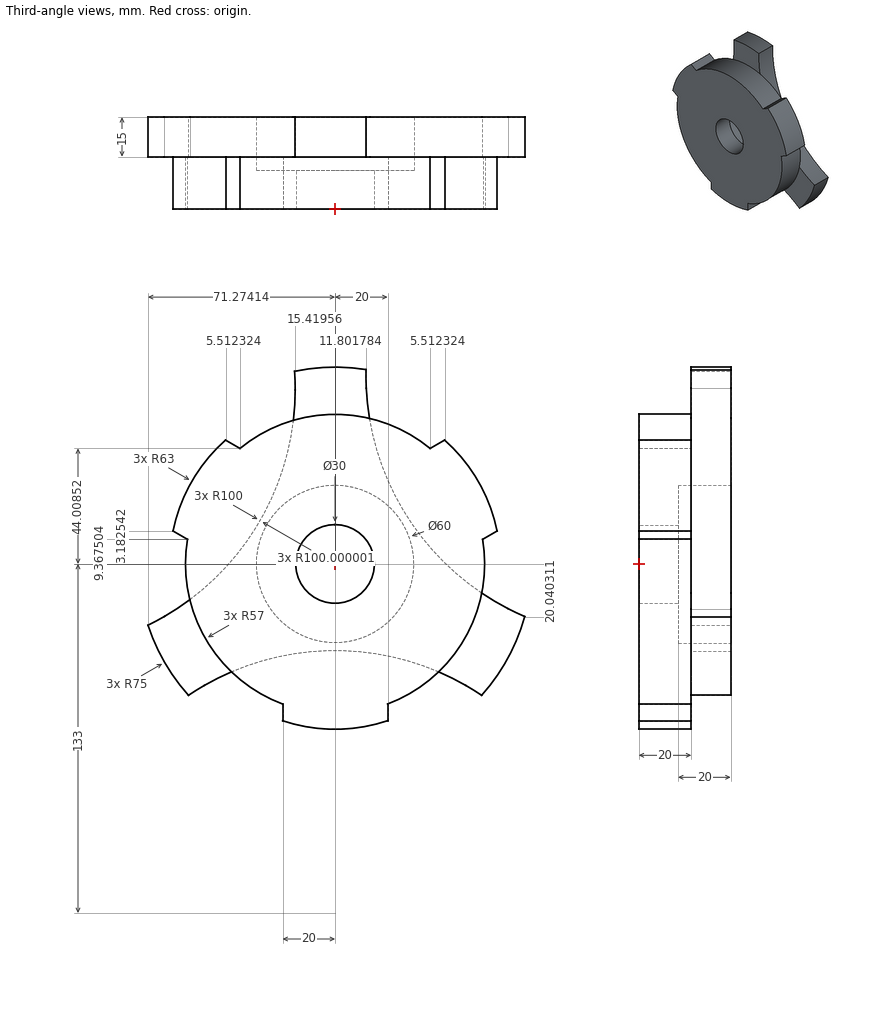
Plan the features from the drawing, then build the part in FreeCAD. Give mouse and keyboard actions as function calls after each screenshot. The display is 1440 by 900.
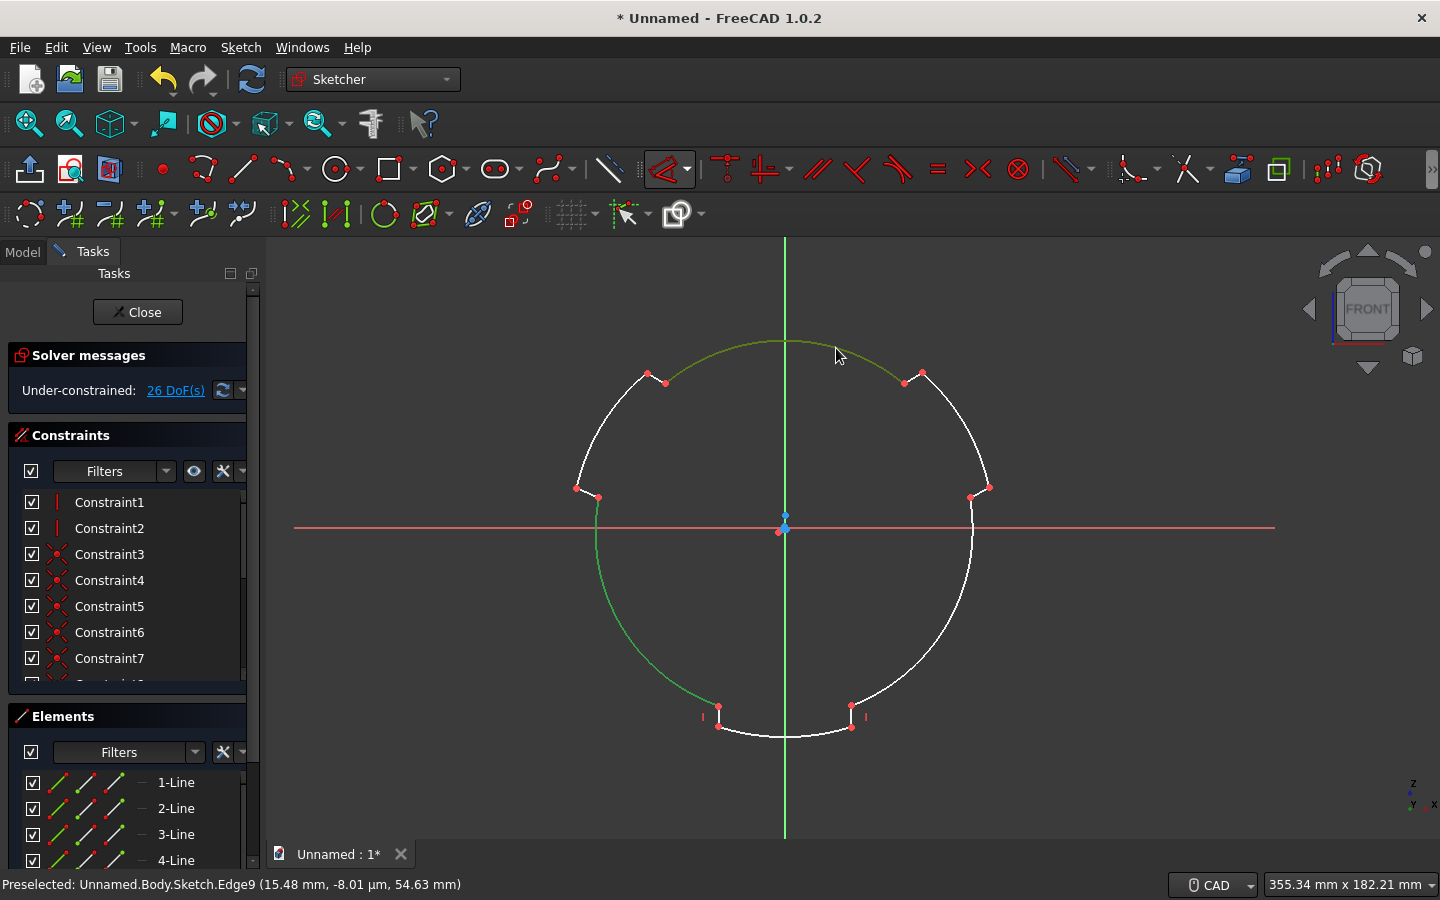
click(726, 170)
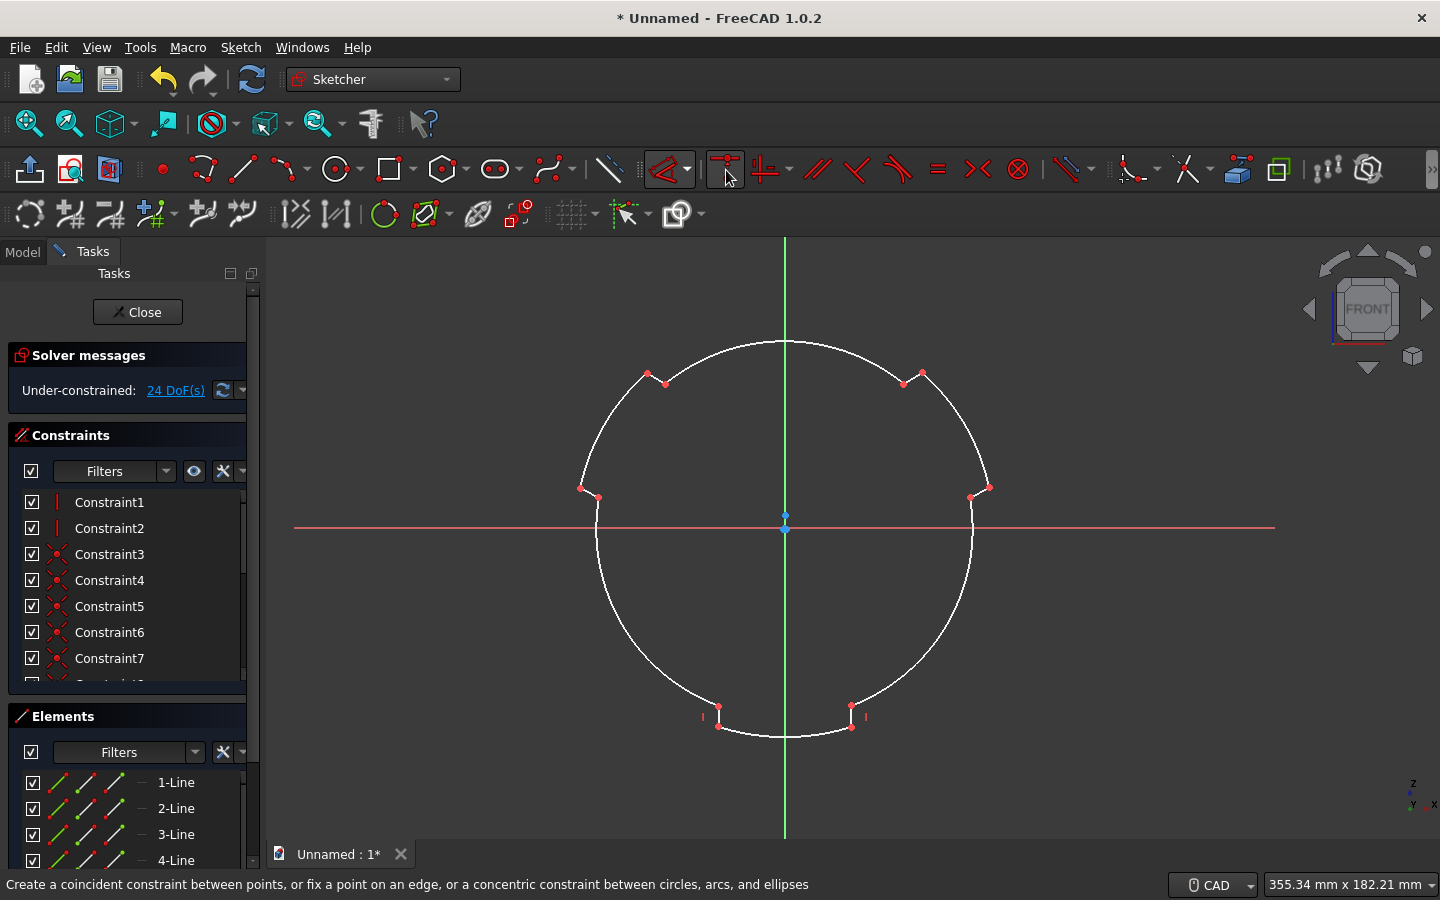
click(602, 576)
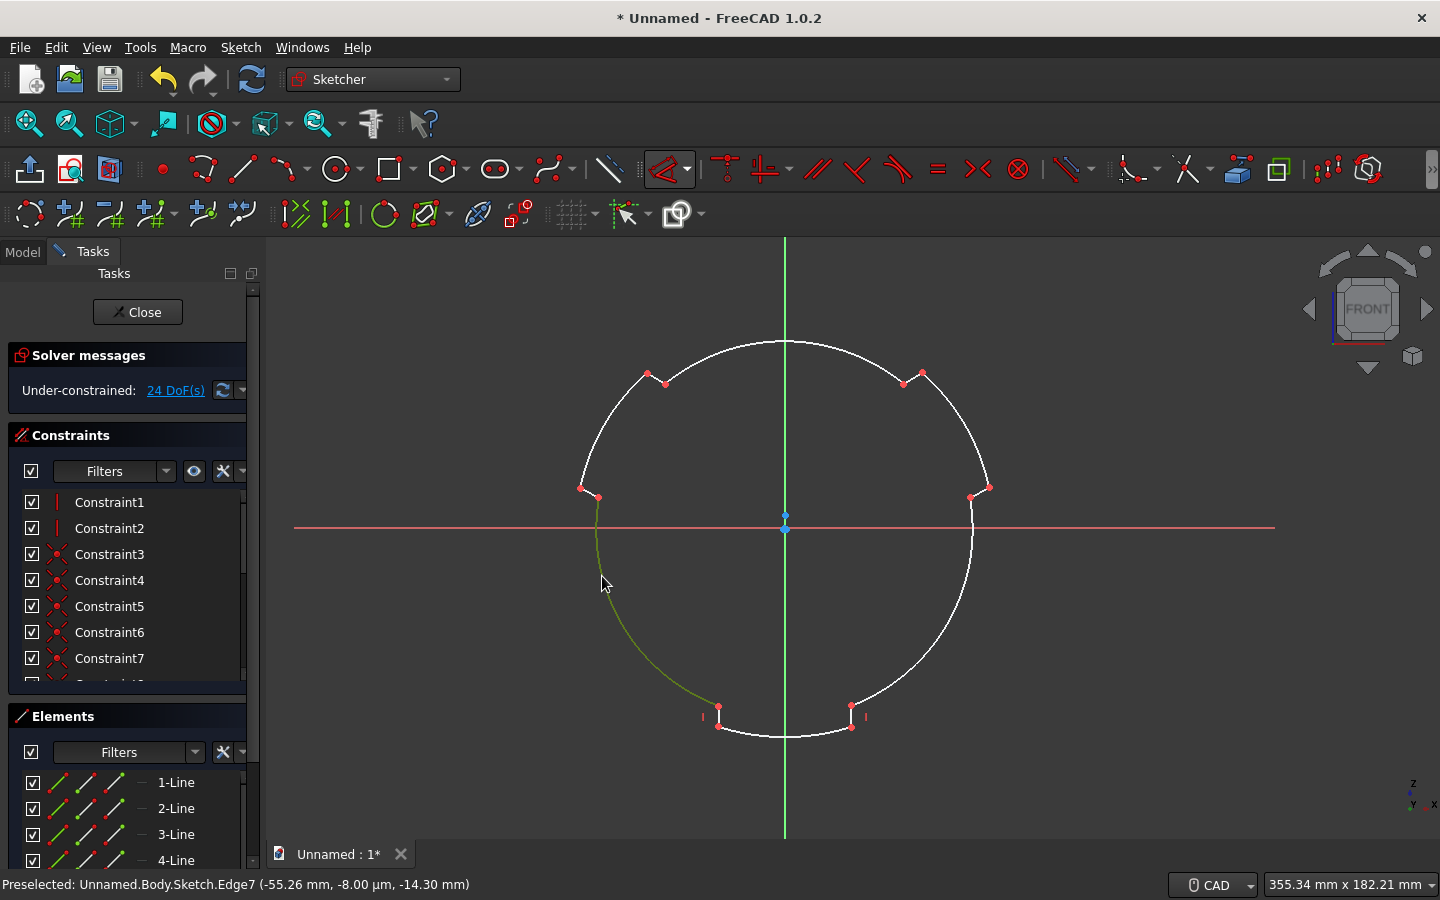
click(977, 449)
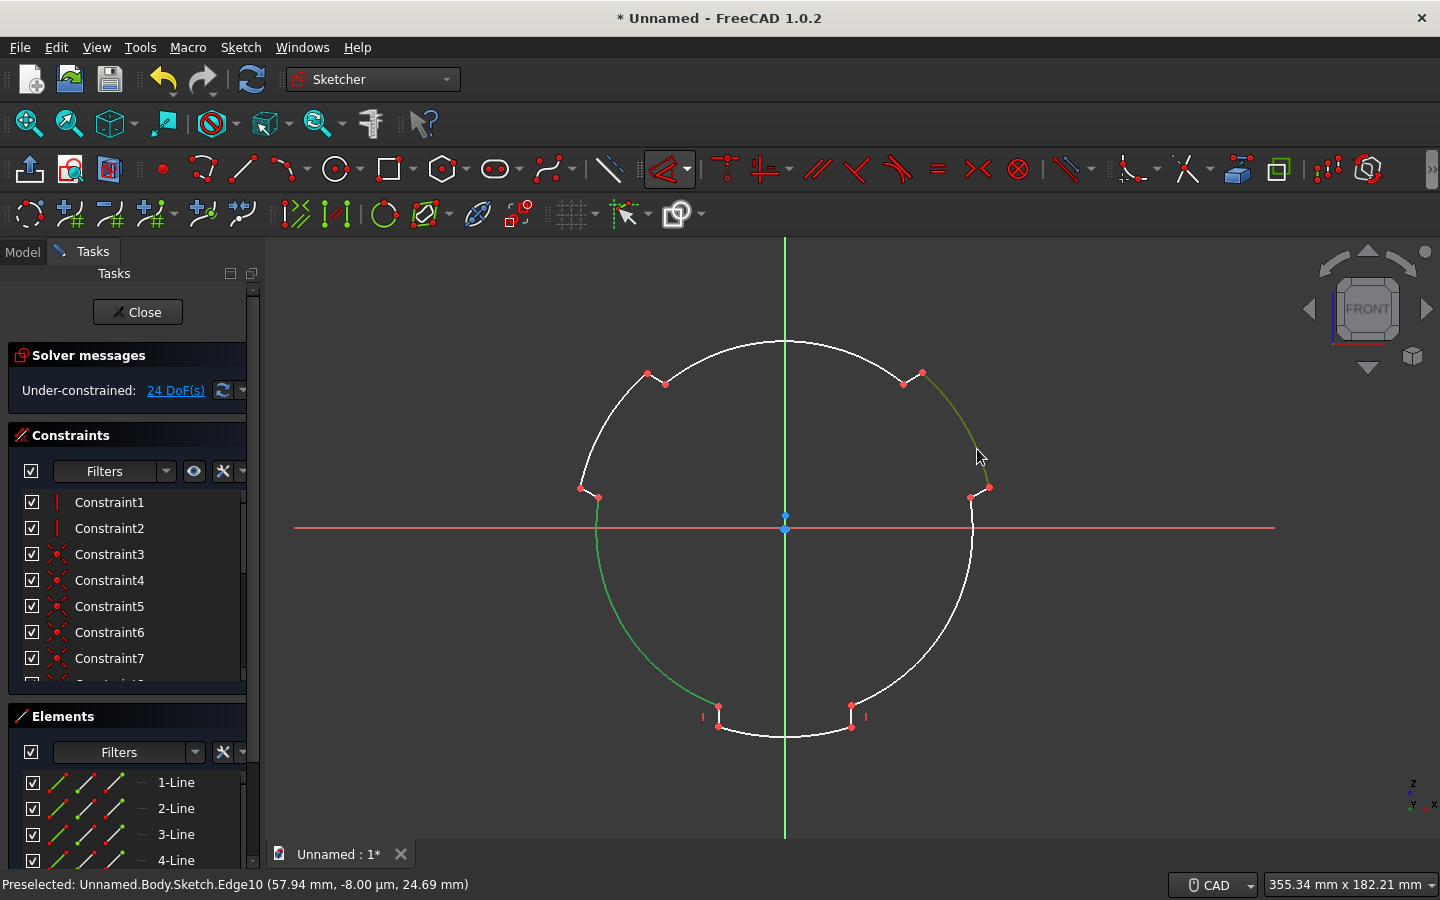
key(c)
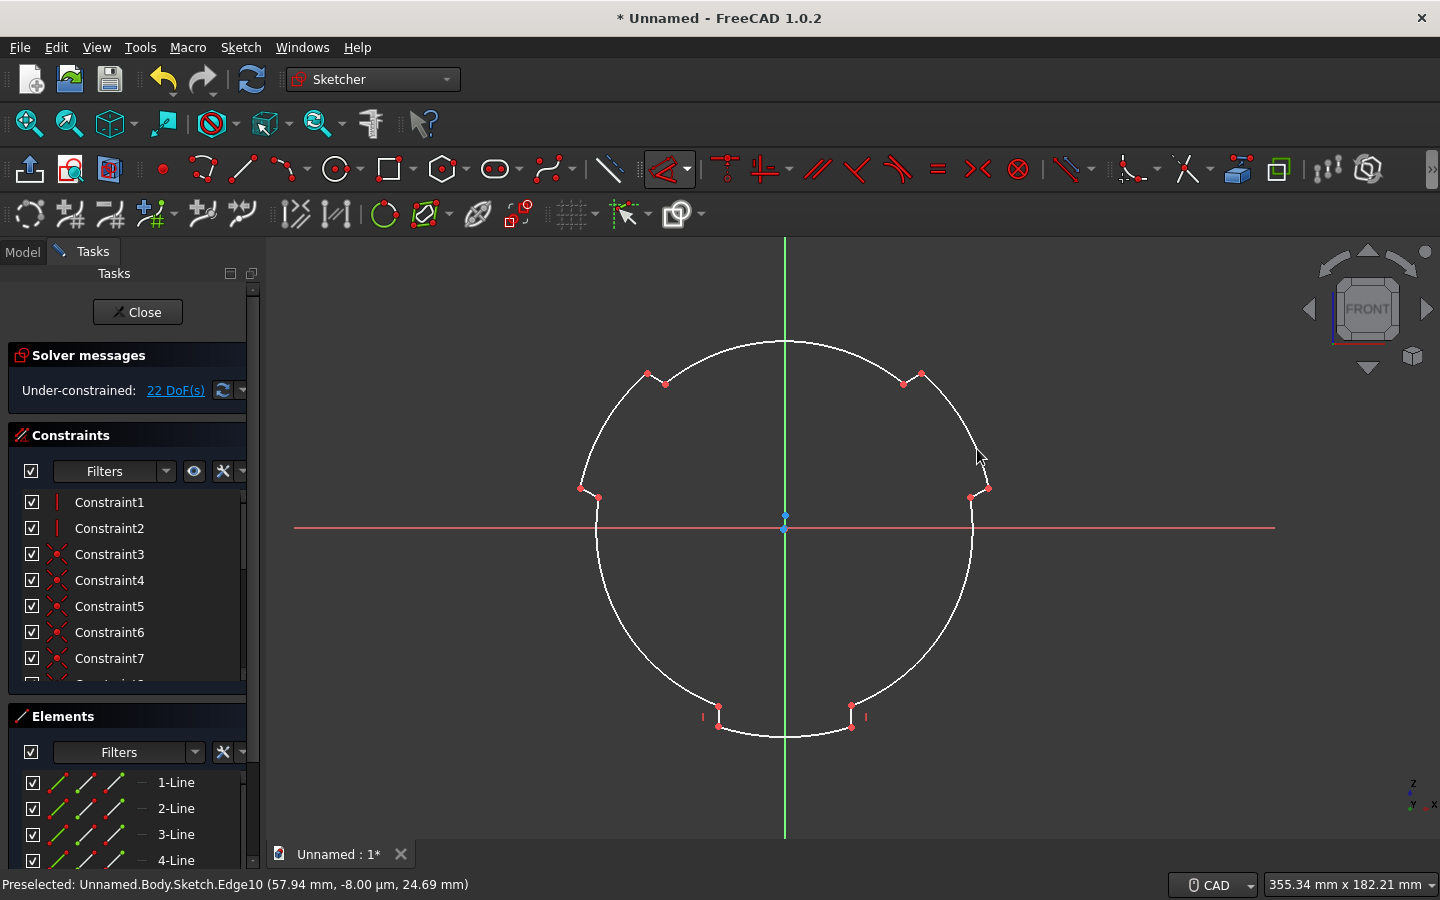
click(602, 576)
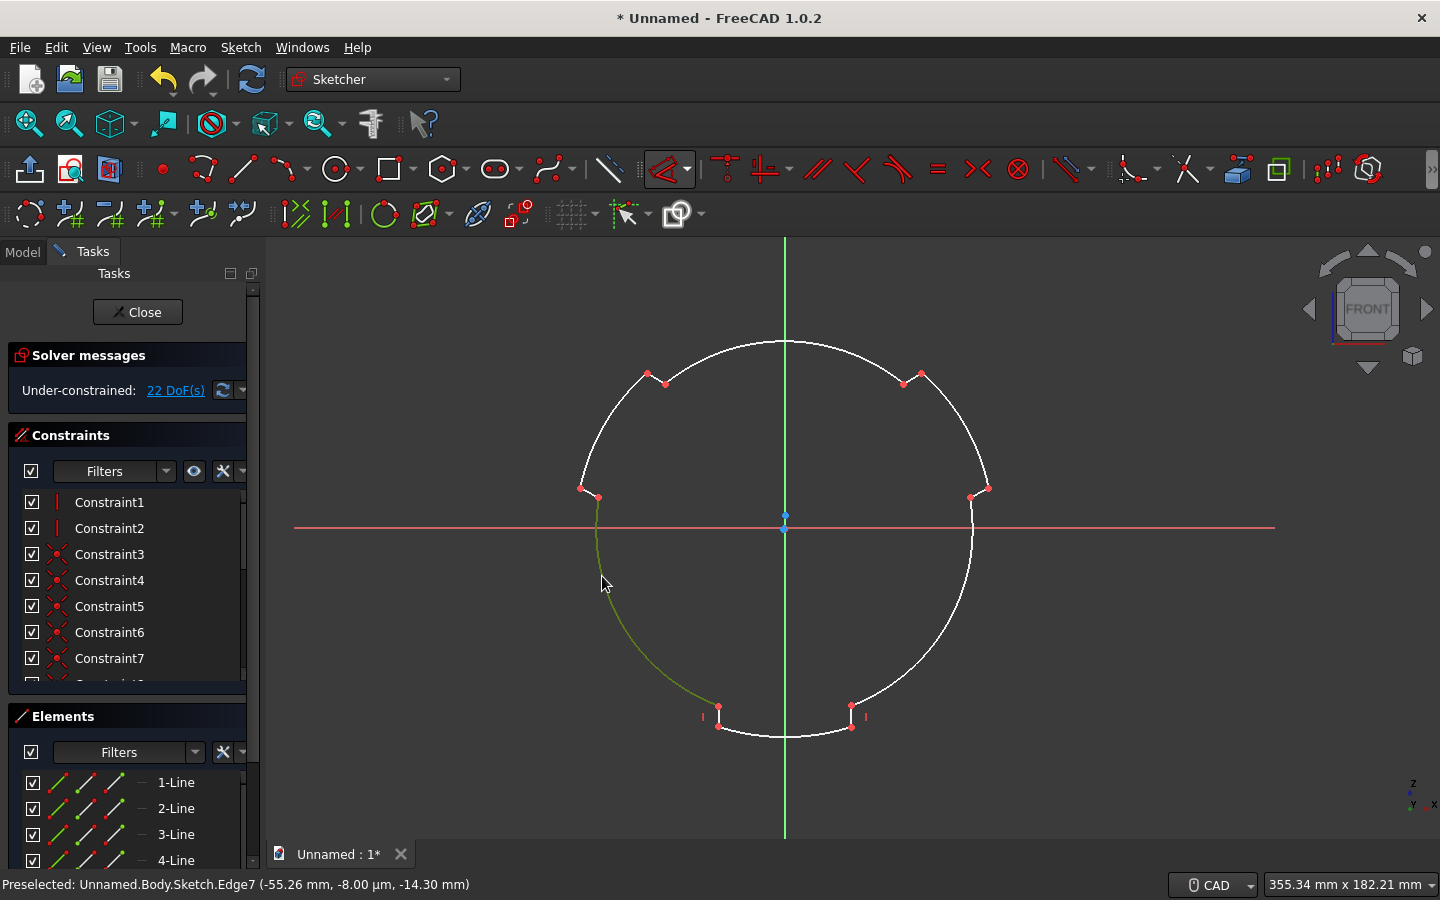
click(916, 664)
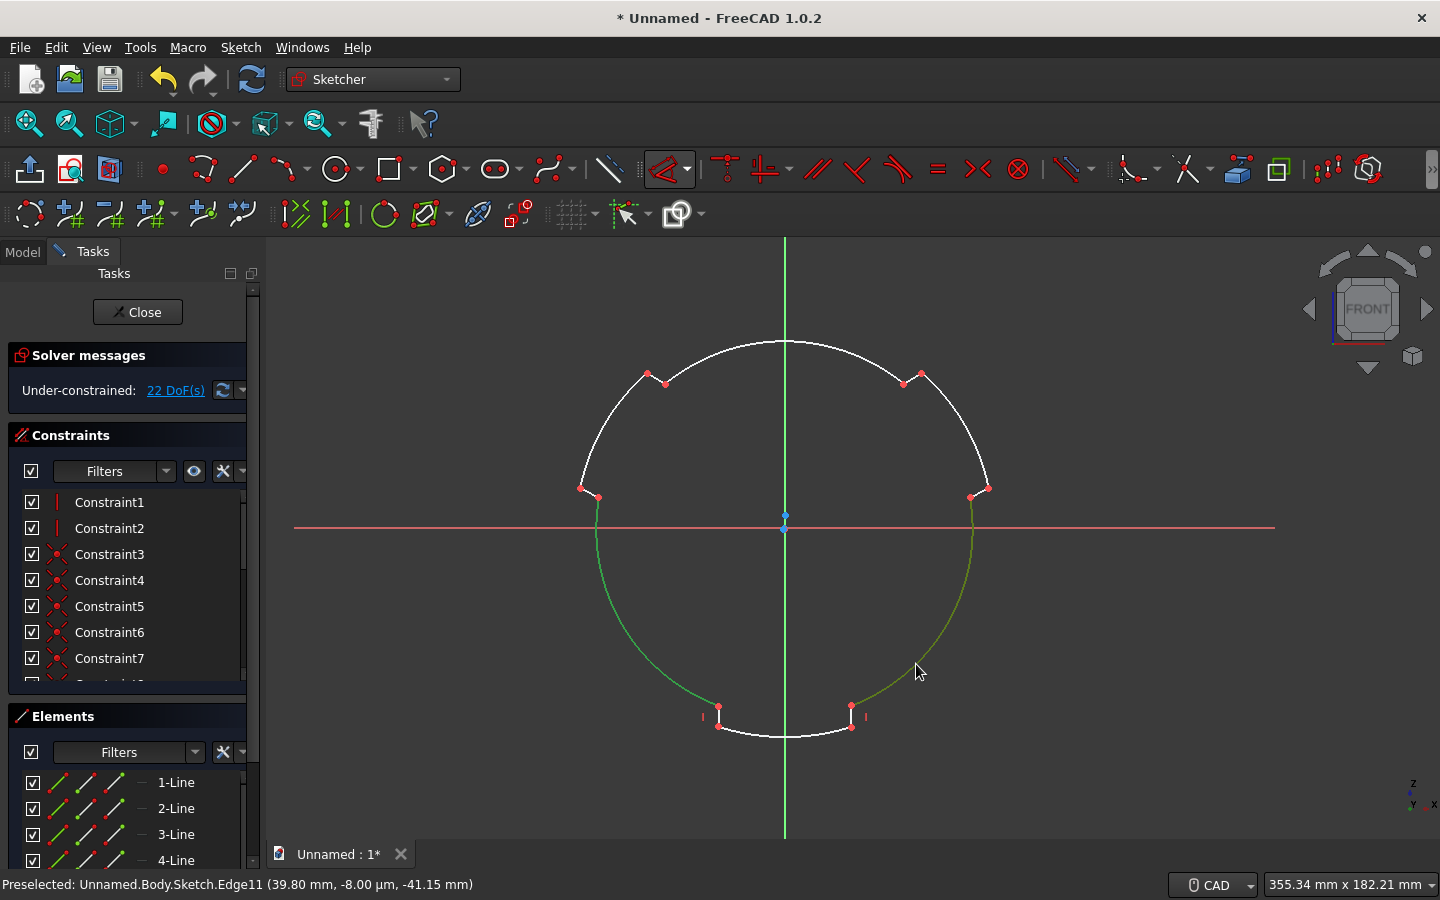
click(726, 170)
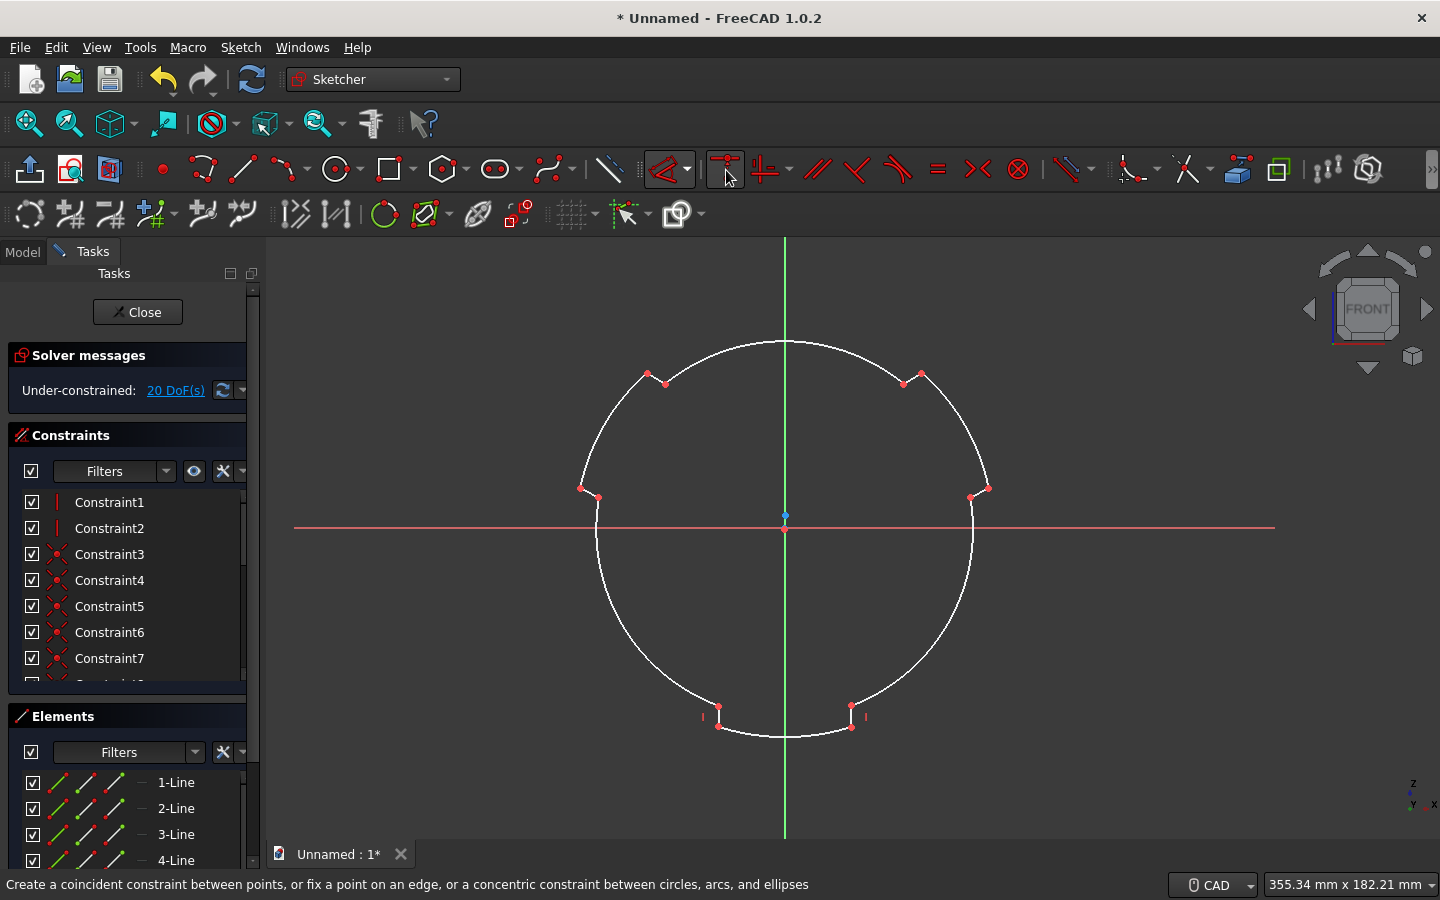
click(602, 576)